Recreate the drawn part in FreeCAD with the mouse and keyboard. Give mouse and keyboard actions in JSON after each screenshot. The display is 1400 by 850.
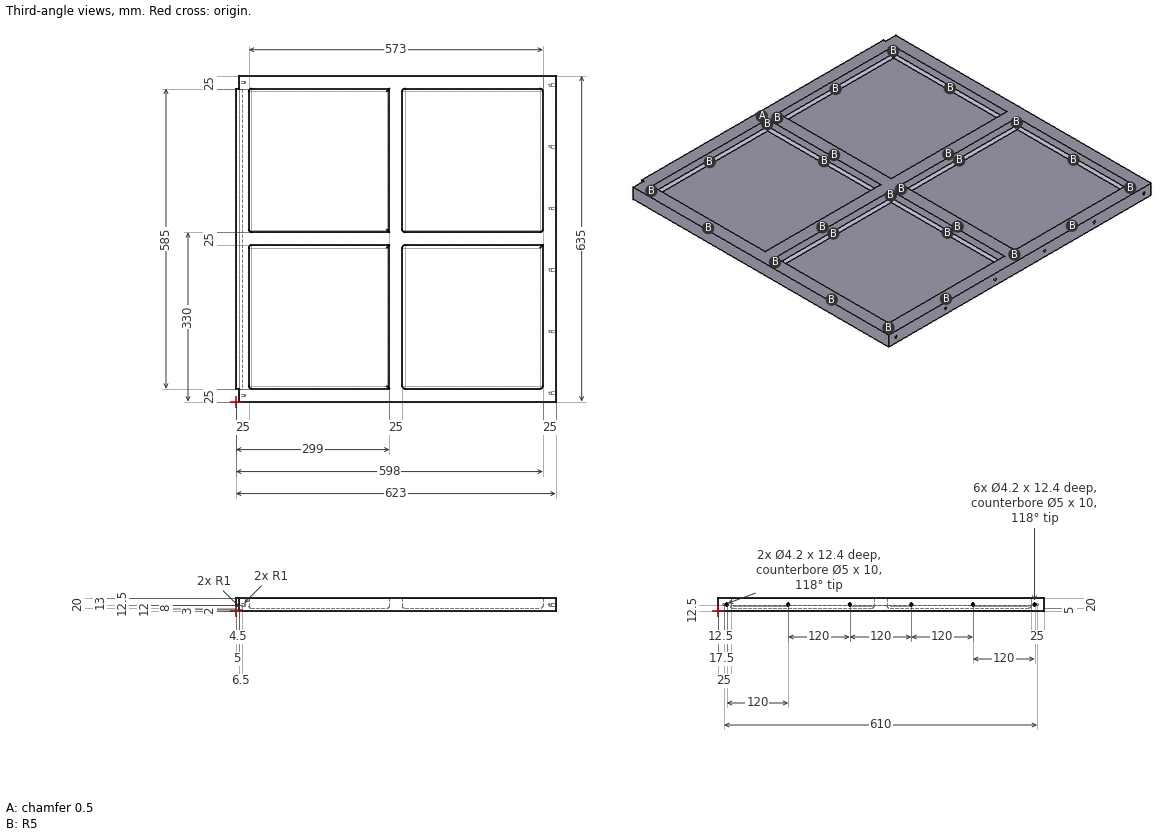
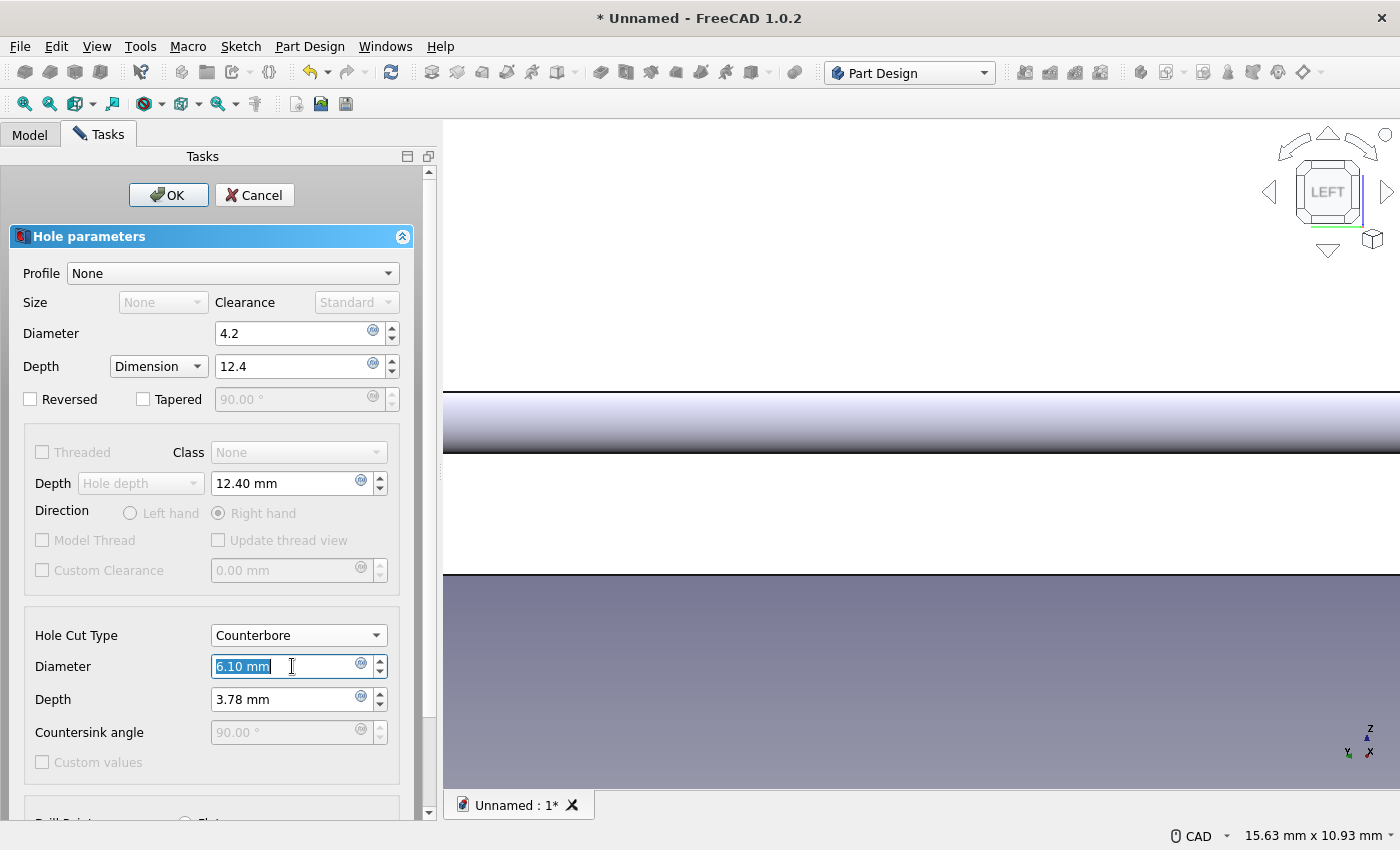
{"action": "type", "text": "5"}
{"action": "key", "text": "Tab"}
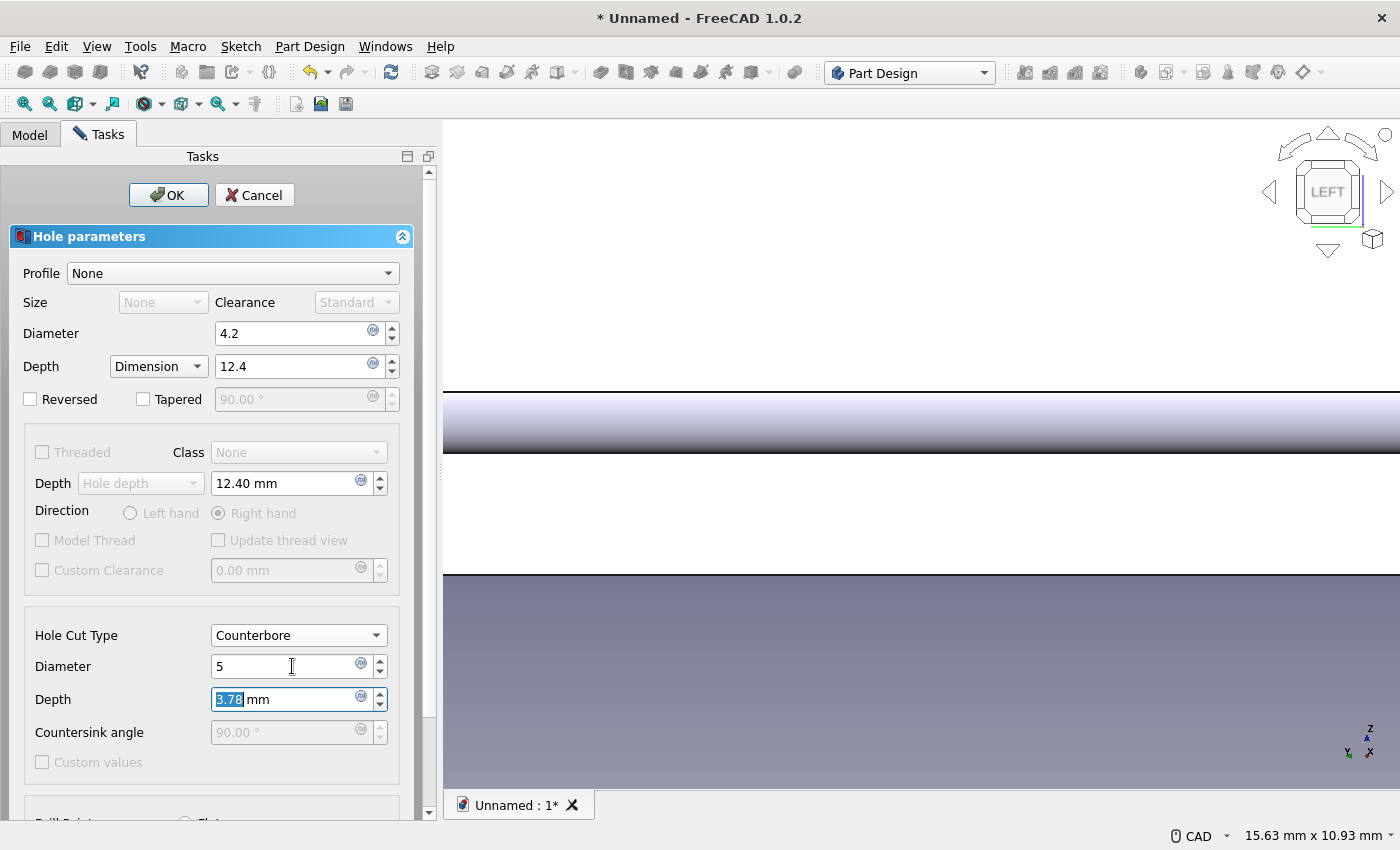
{"action": "type", "text": "10"}
{"action": "key", "text": "Tab"}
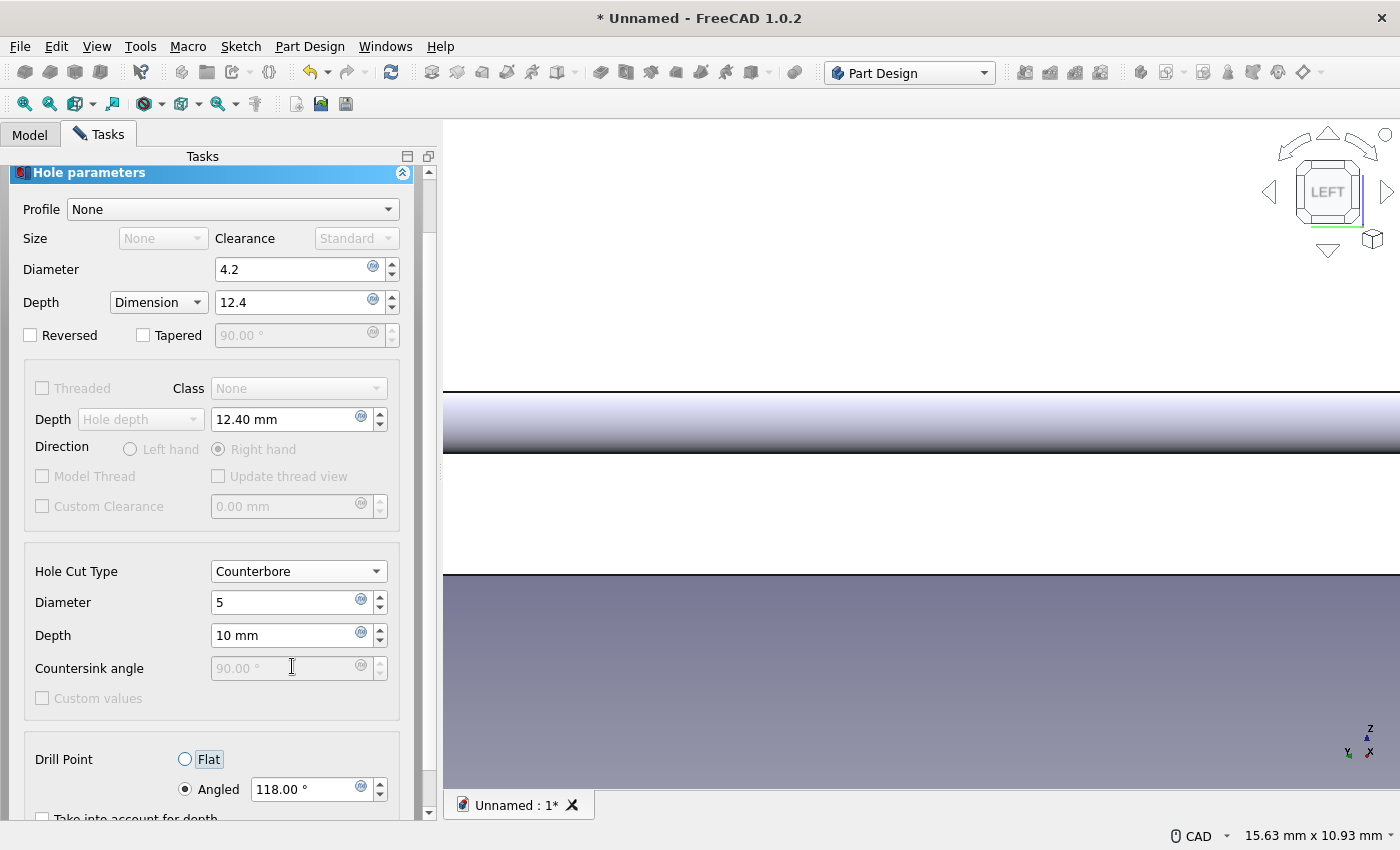
{"action": "scroll", "coordinate": [429, 493], "scroll_direction": "up", "scroll_amount": 2}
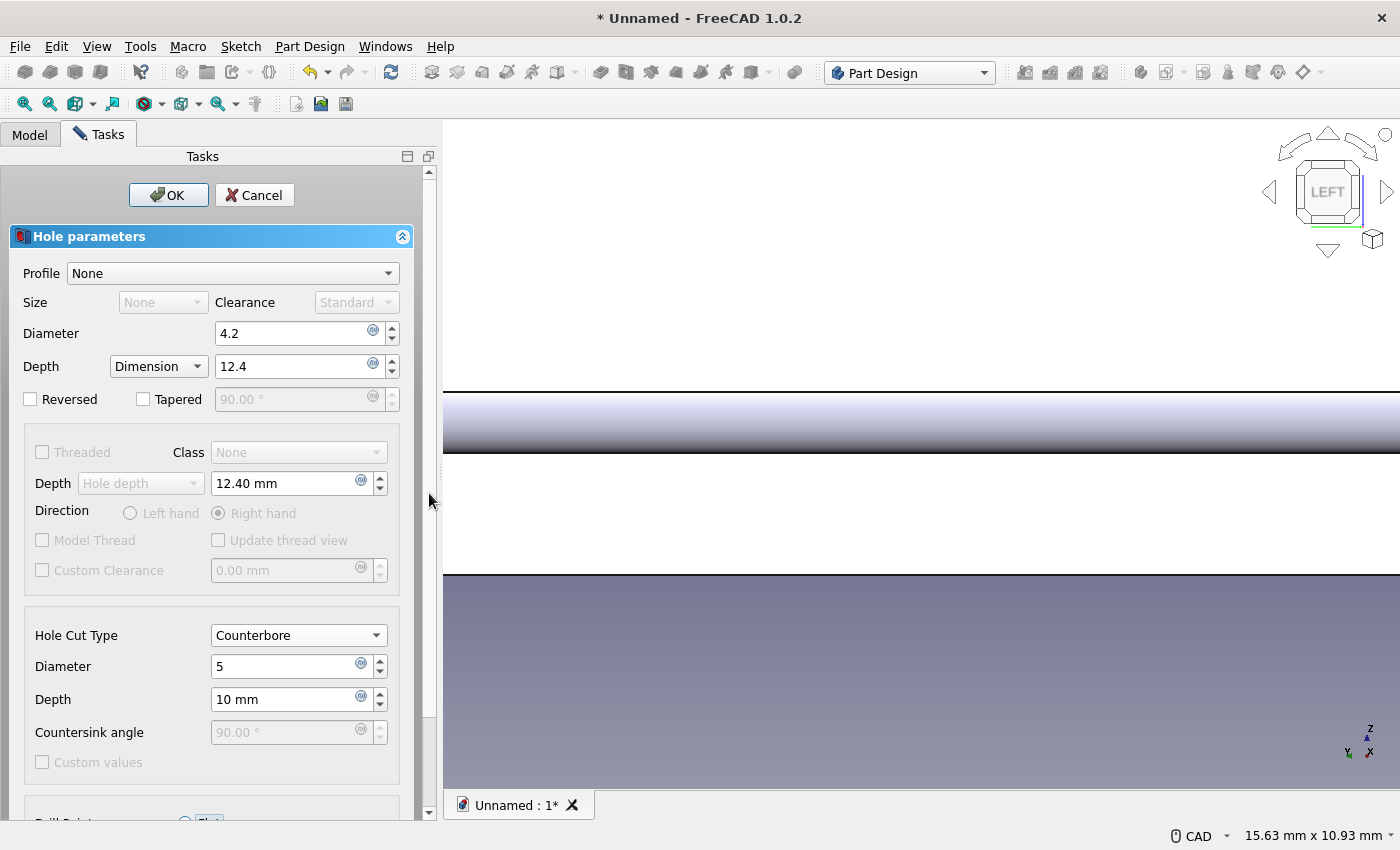
{"action": "left_click", "coordinate": [169, 195]}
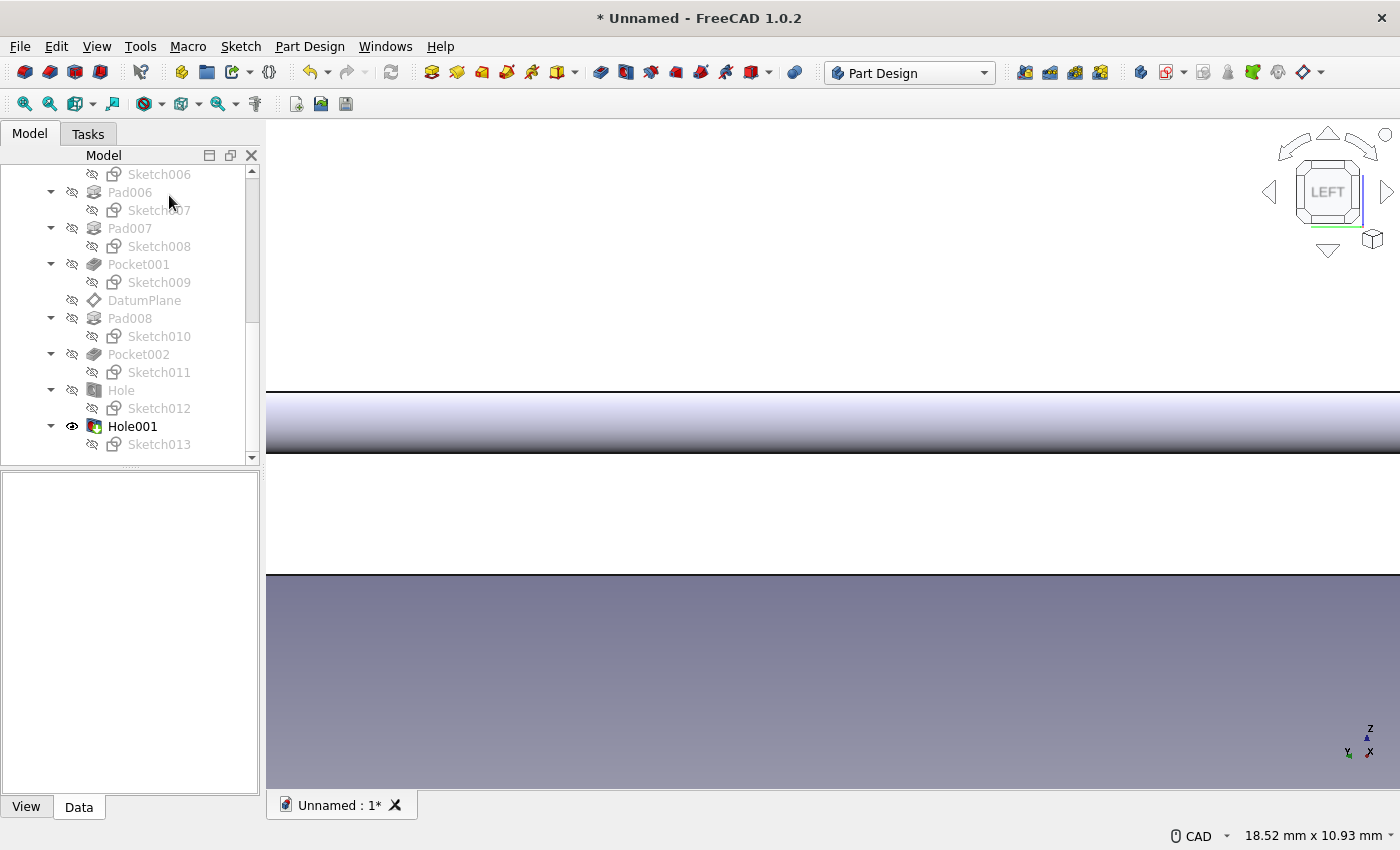
{"action": "left_click", "coordinate": [25, 104]}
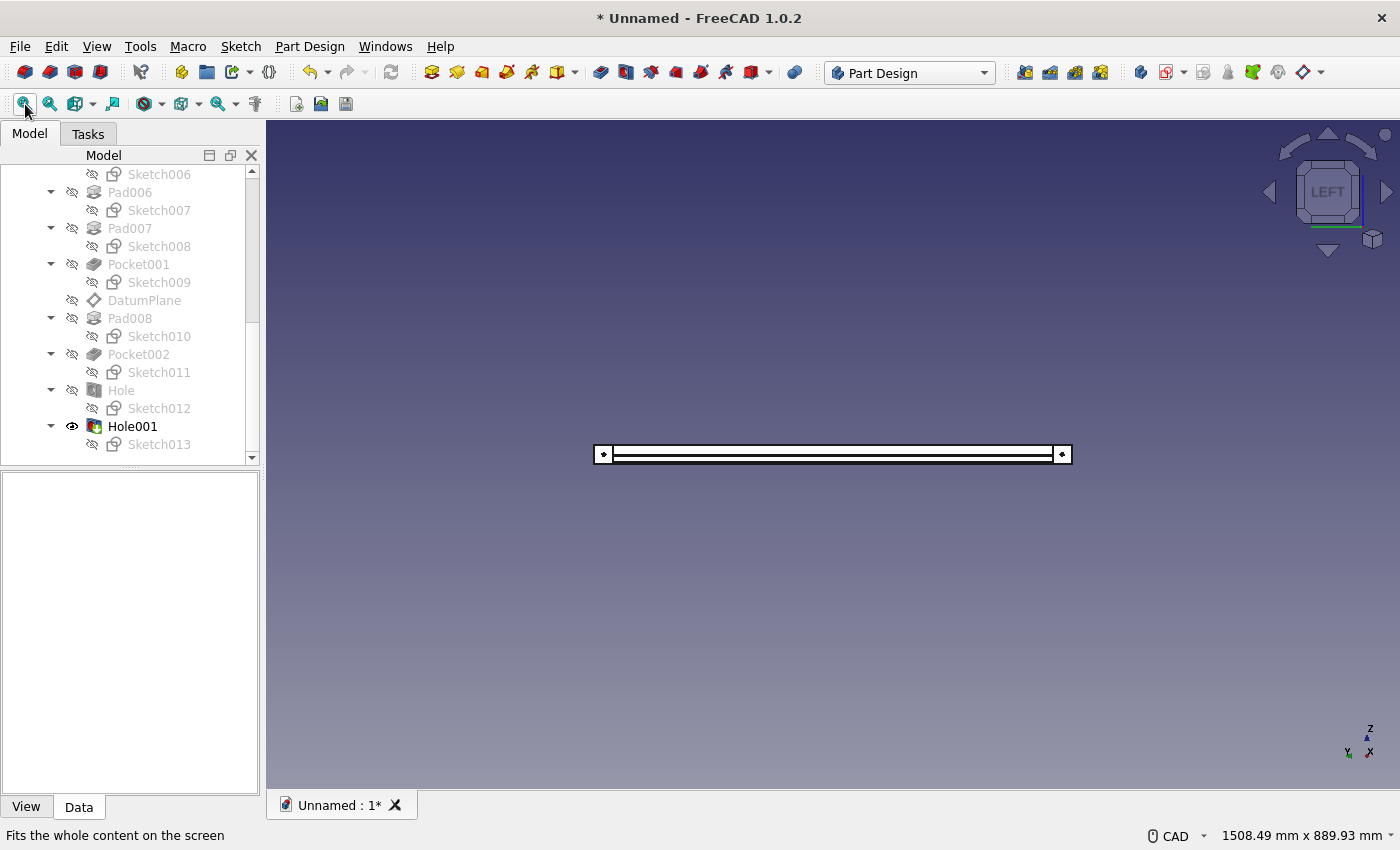
{"action": "key", "text": "0"}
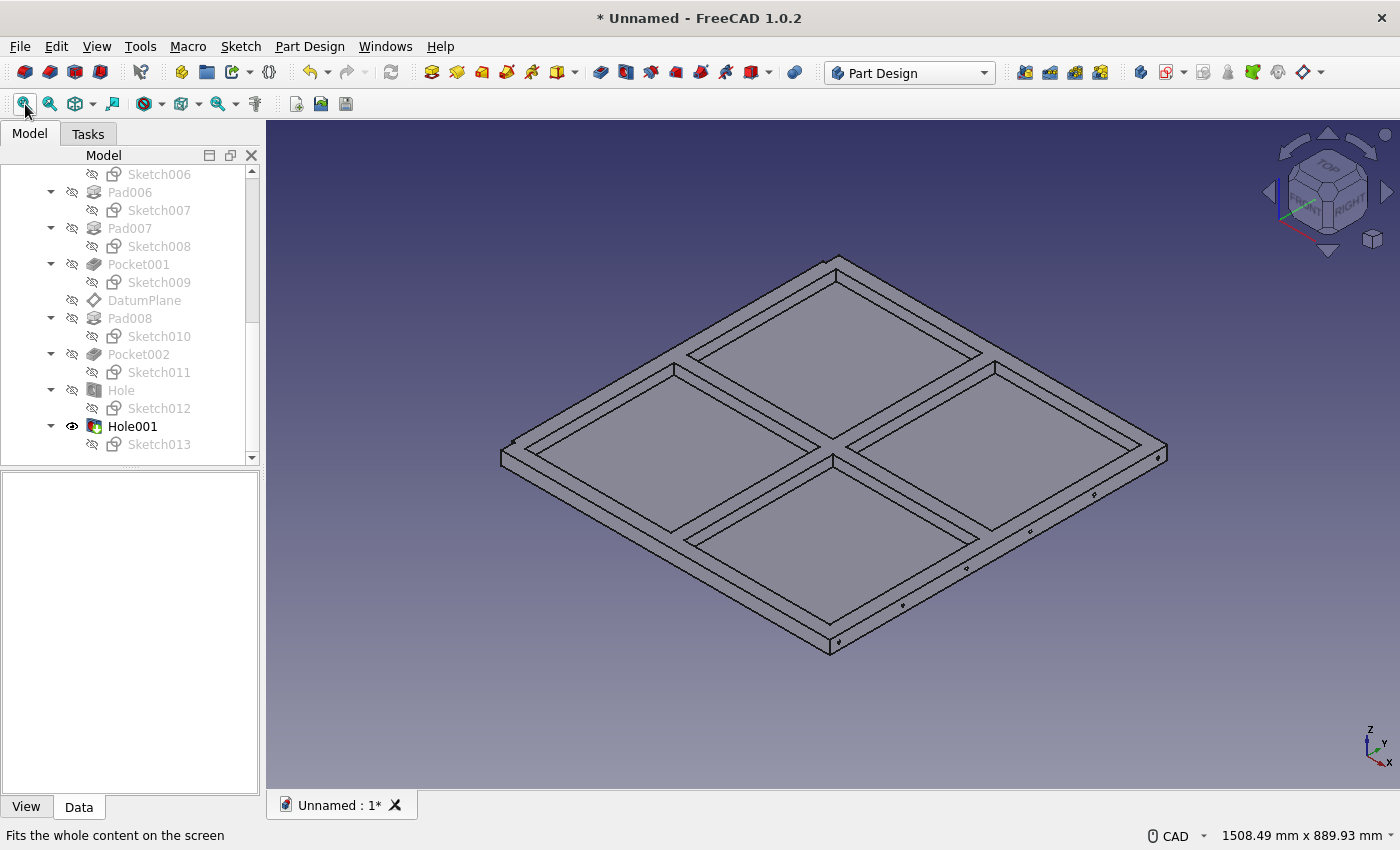
{"action": "left_click", "coordinate": [672, 459]}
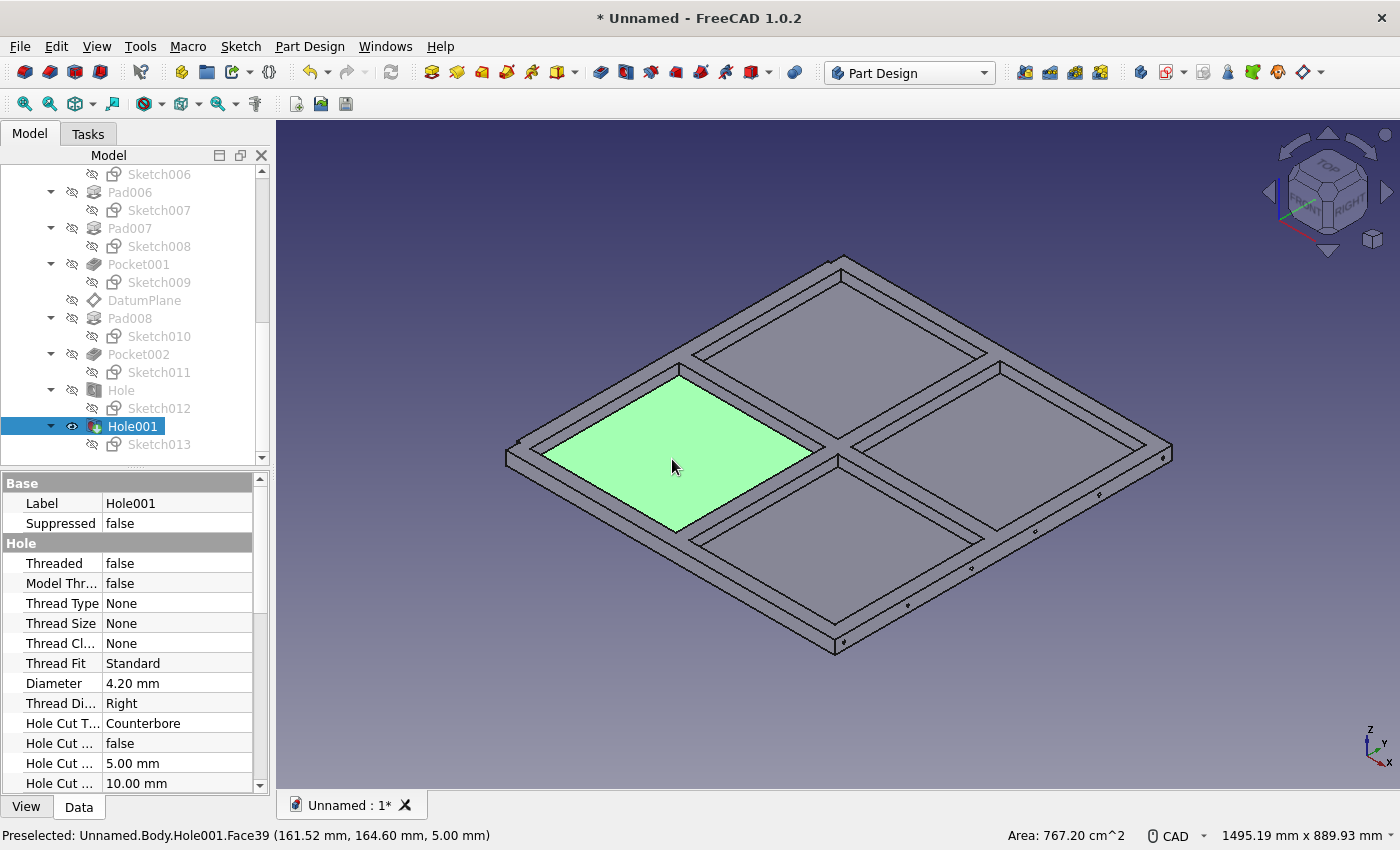
{"action": "left_click", "coordinate": [836, 551], "text": "ctrl"}